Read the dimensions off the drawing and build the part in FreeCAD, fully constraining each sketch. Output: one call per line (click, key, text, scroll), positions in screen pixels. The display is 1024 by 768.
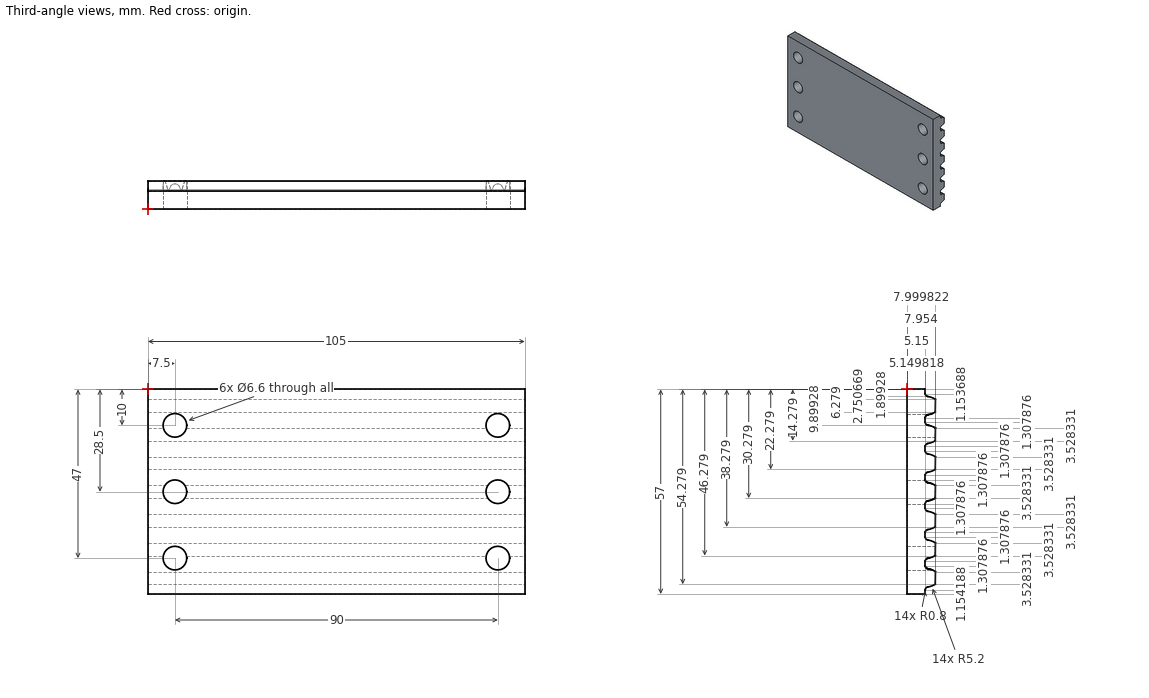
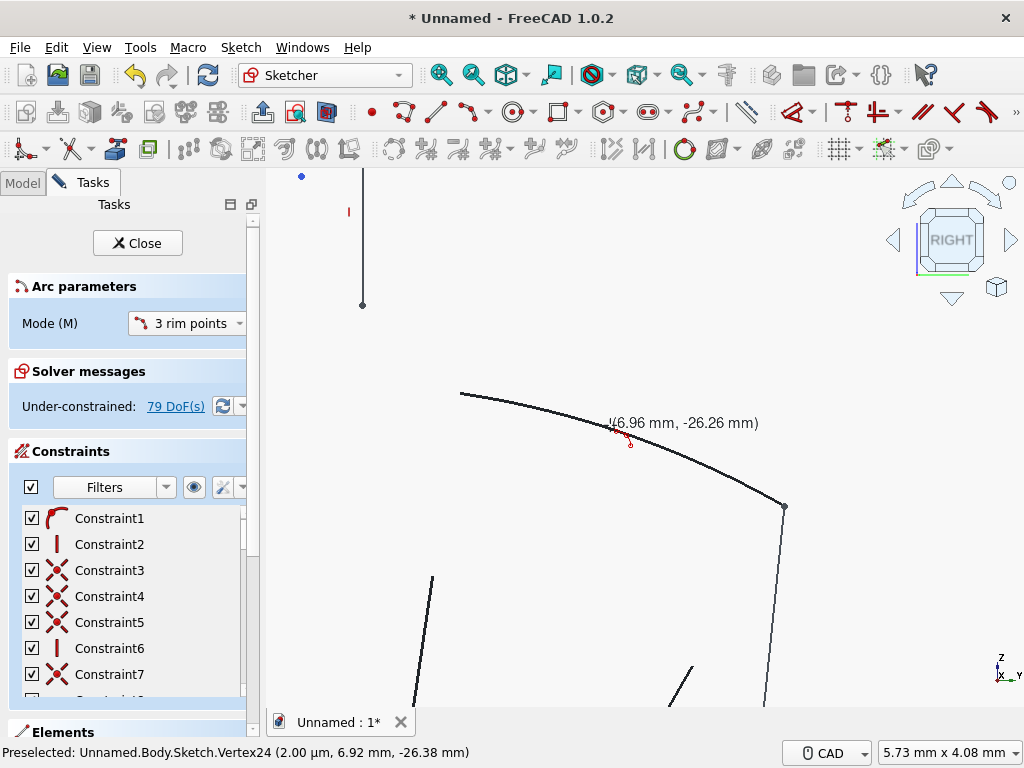
click(609, 423)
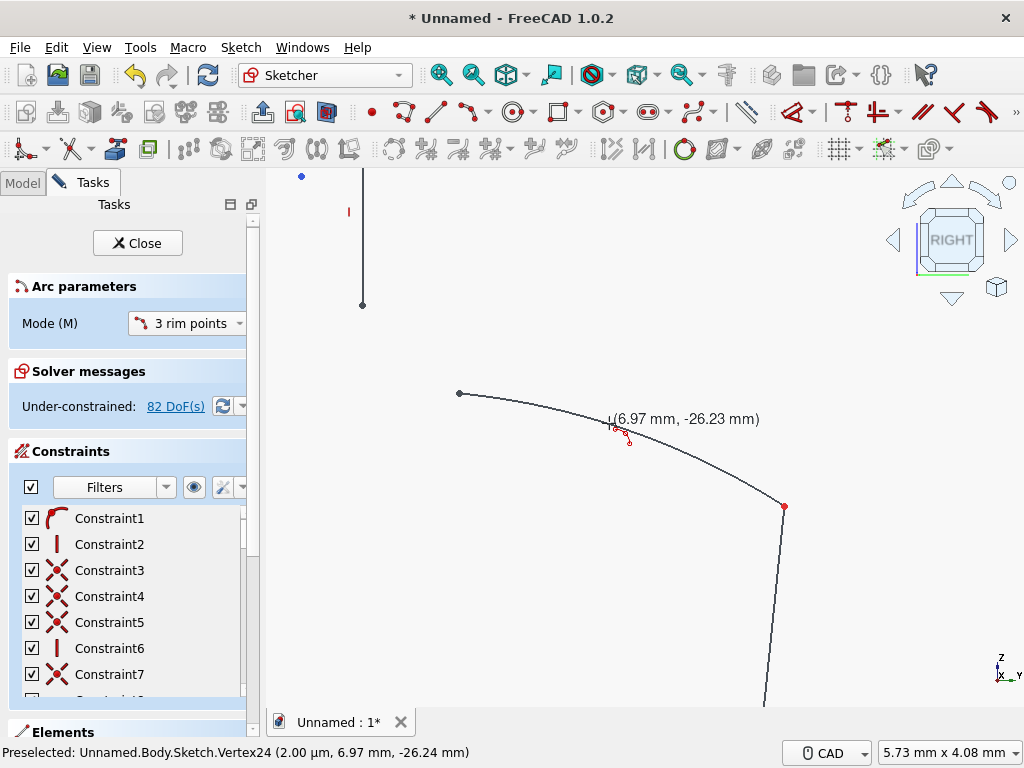
scroll(595, 423, down, 15)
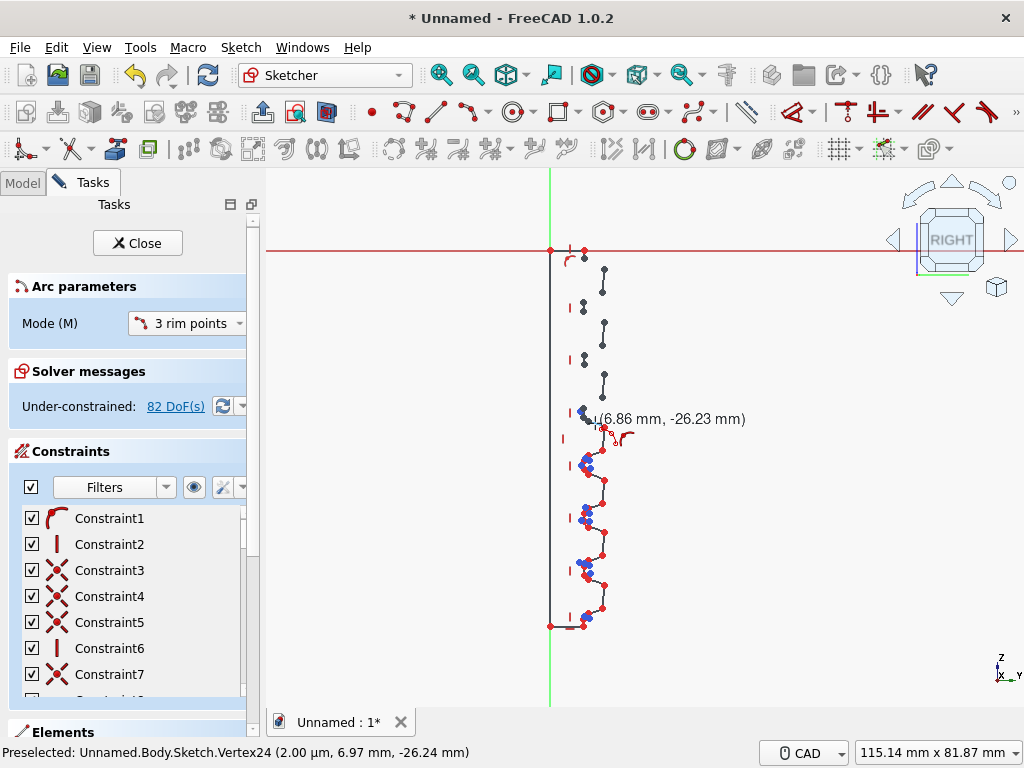
scroll(589, 422, up, 7)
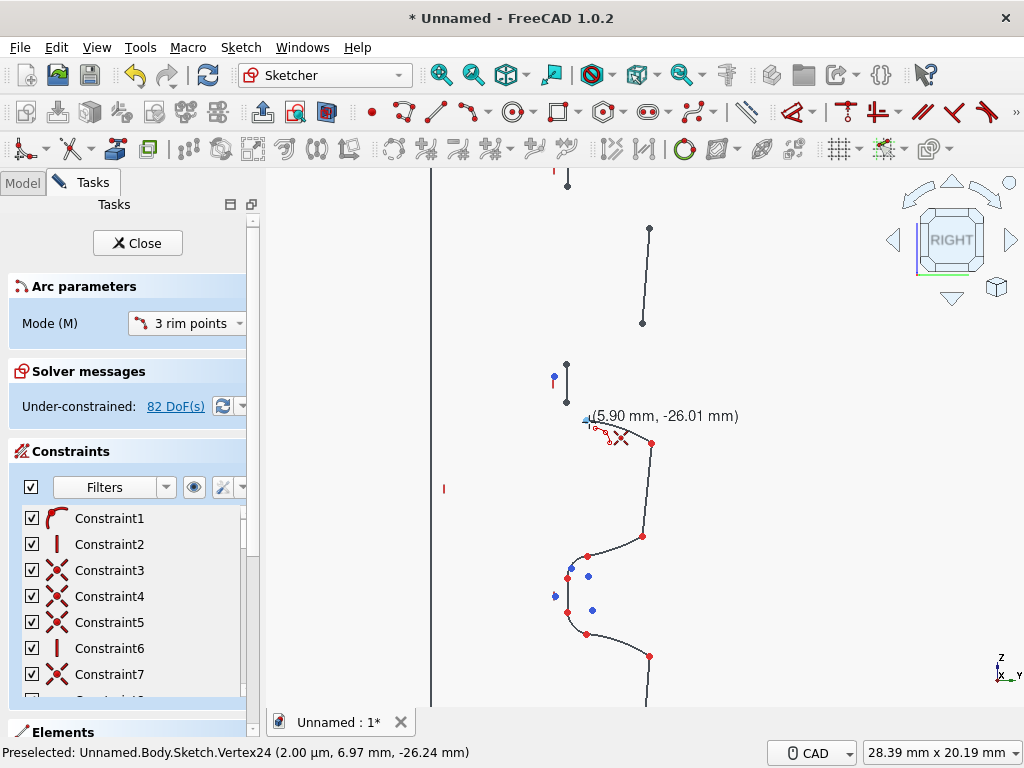
click(586, 420)
click(567, 403)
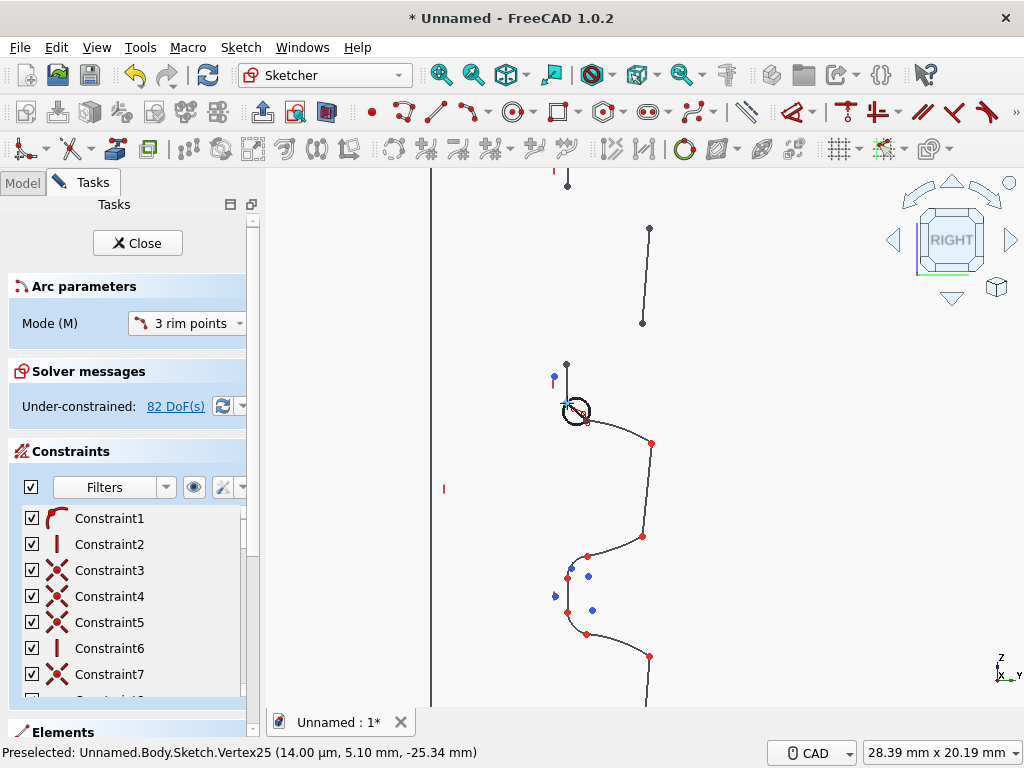
scroll(573, 412, up, 6)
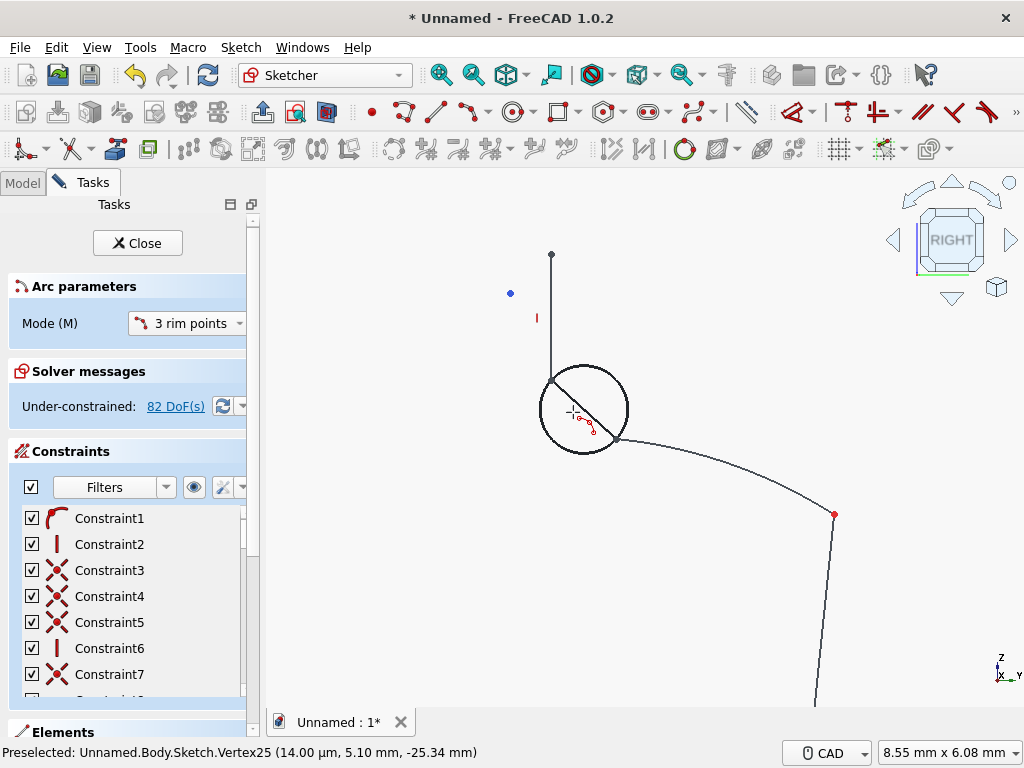
click(573, 411)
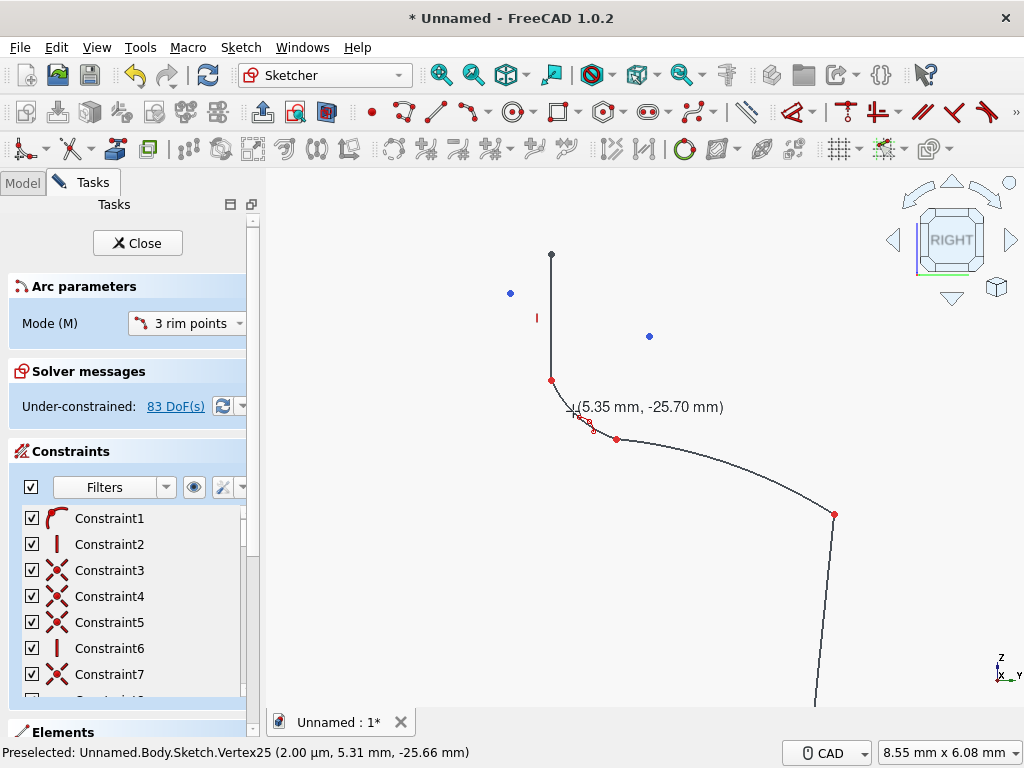
scroll(586, 420, down, 13)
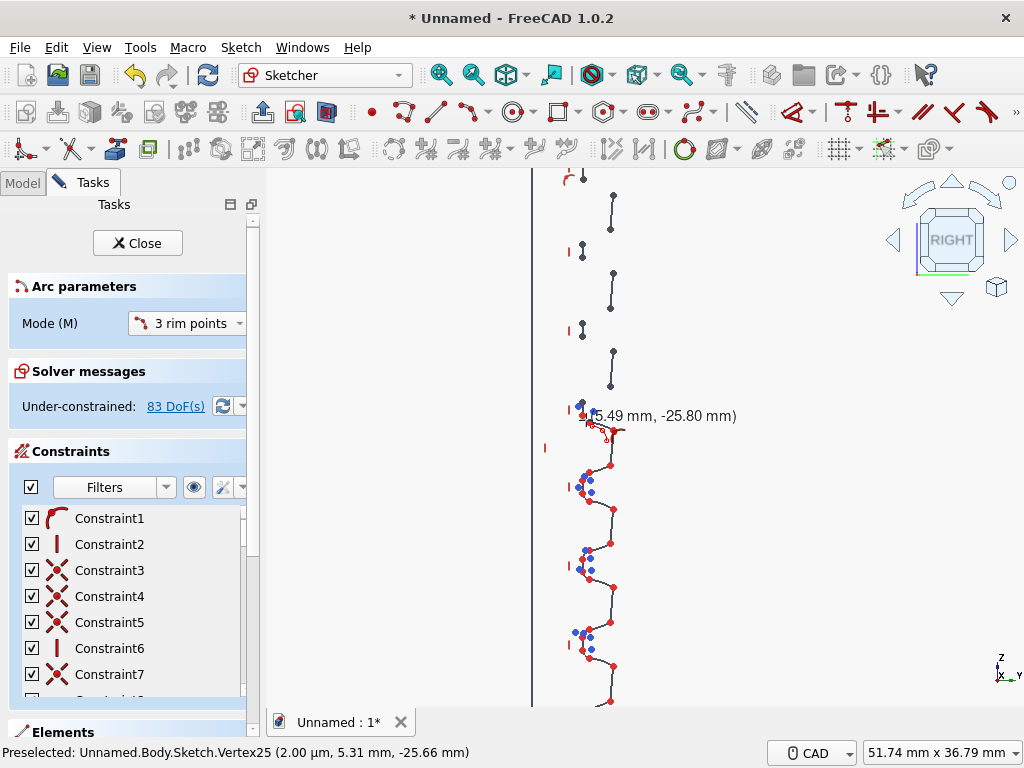
scroll(584, 408, up, 7)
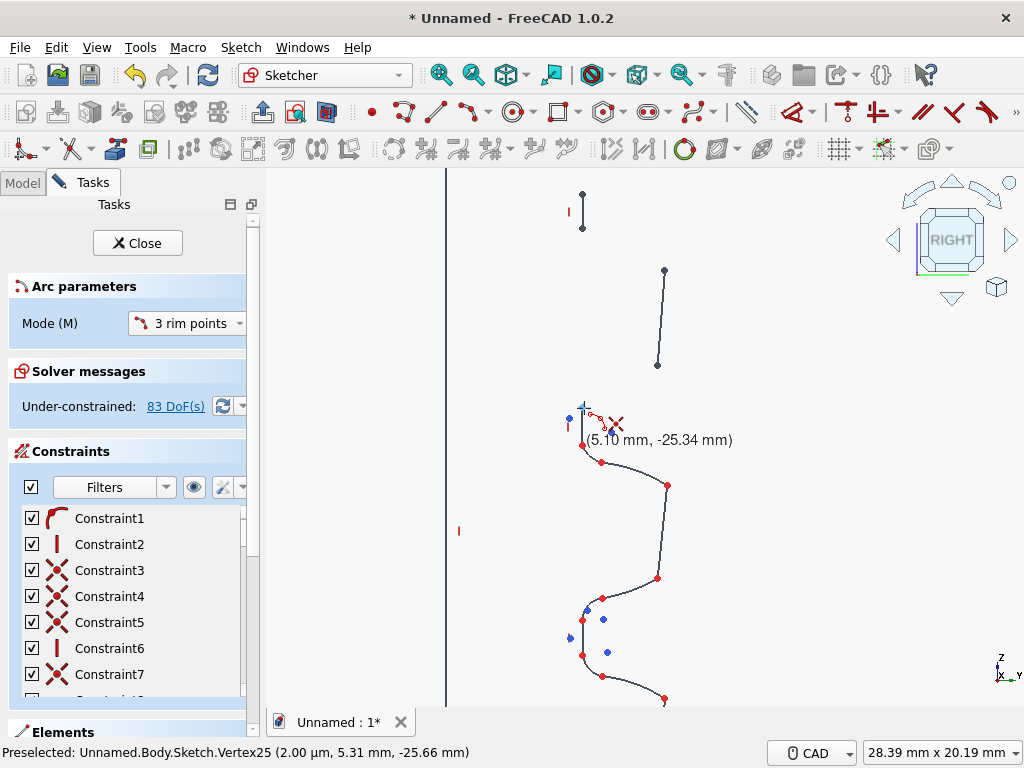
click(582, 407)
click(602, 384)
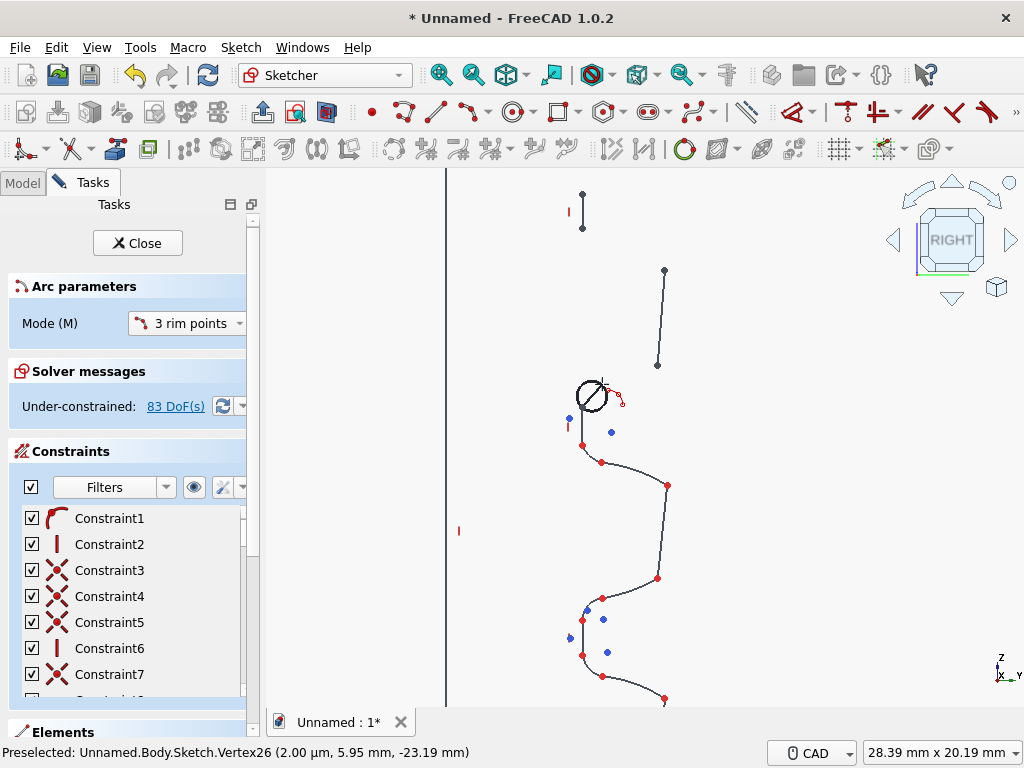
scroll(589, 391, up, 6)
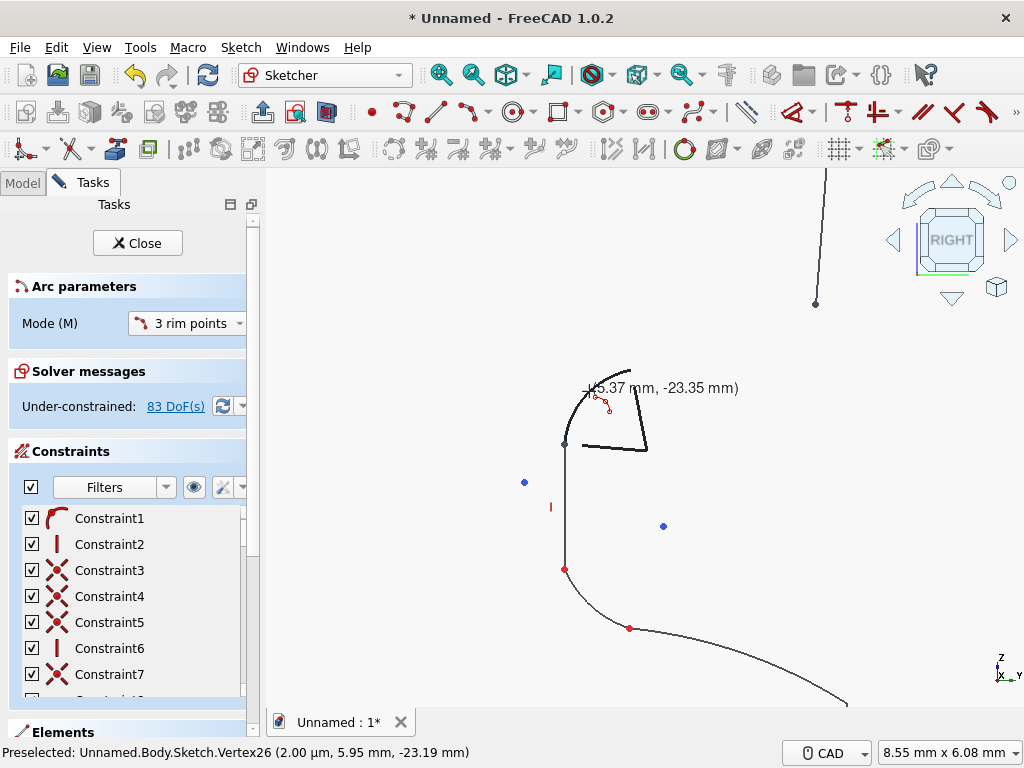
click(586, 391)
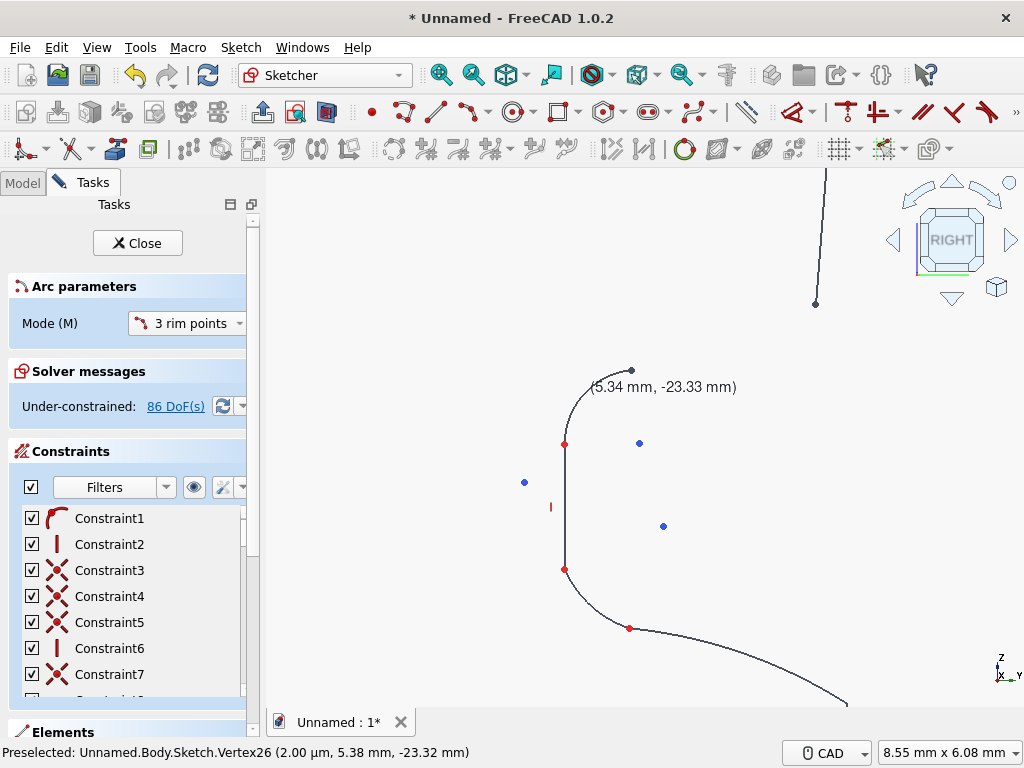
scroll(585, 404, down, 13)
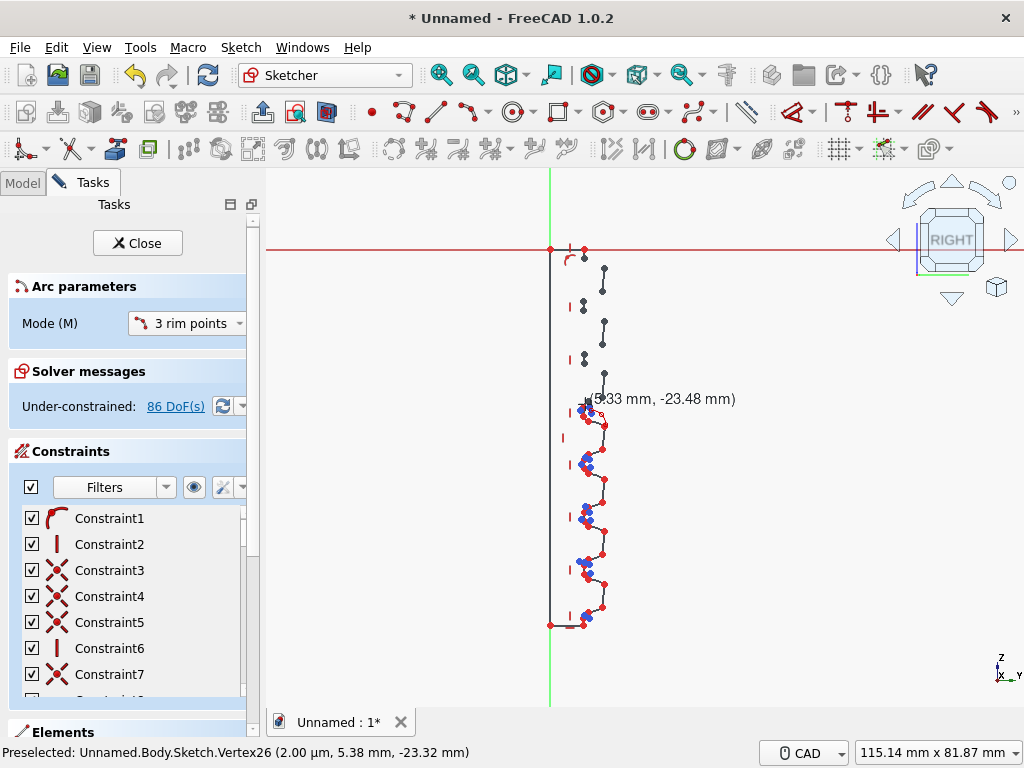
scroll(589, 402, up, 6)